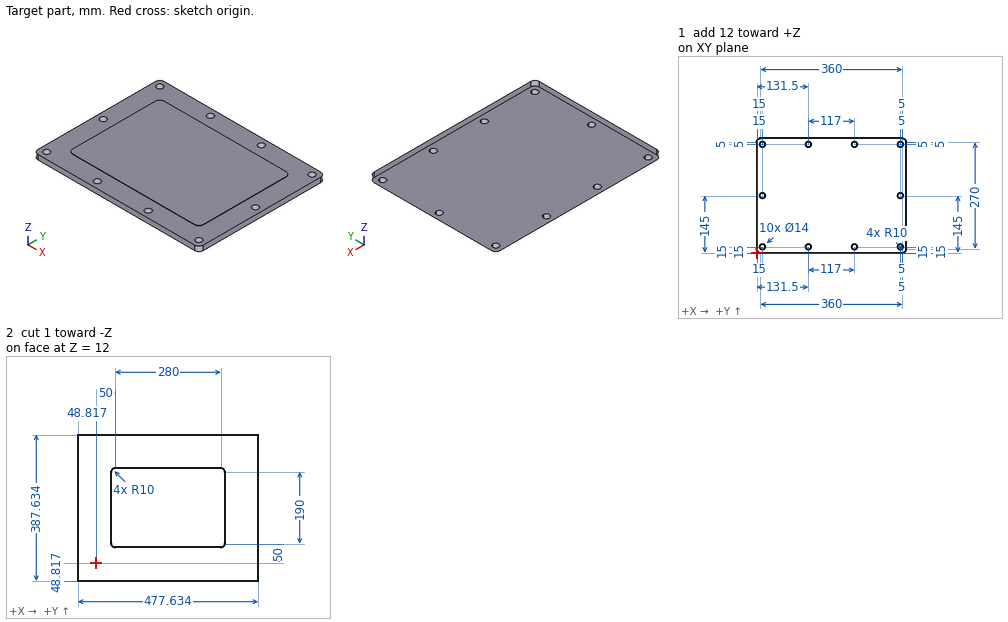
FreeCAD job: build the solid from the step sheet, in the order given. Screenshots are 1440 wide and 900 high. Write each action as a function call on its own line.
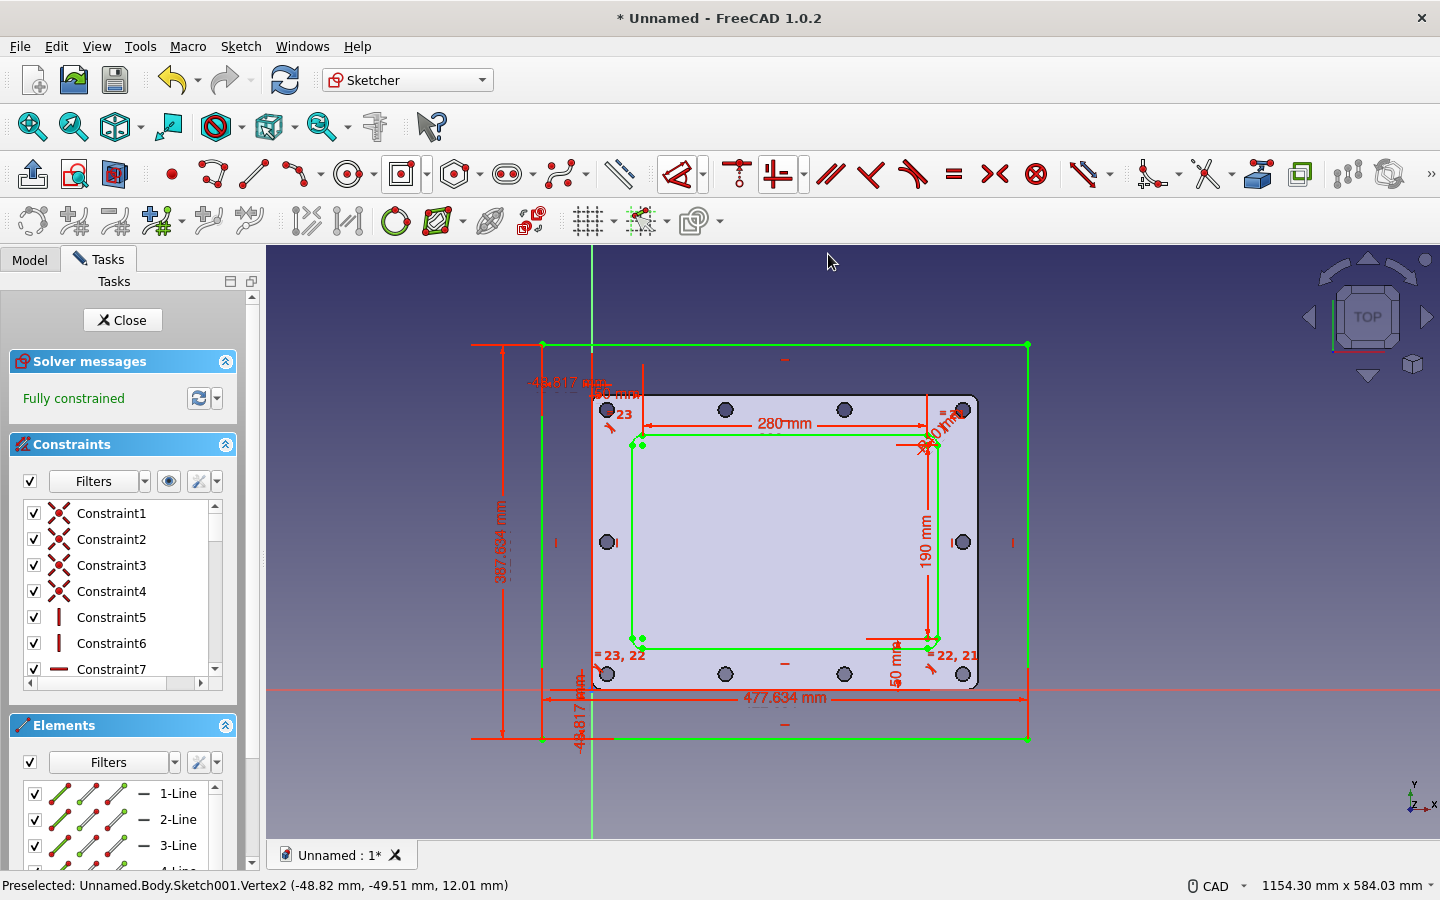
click(123, 320)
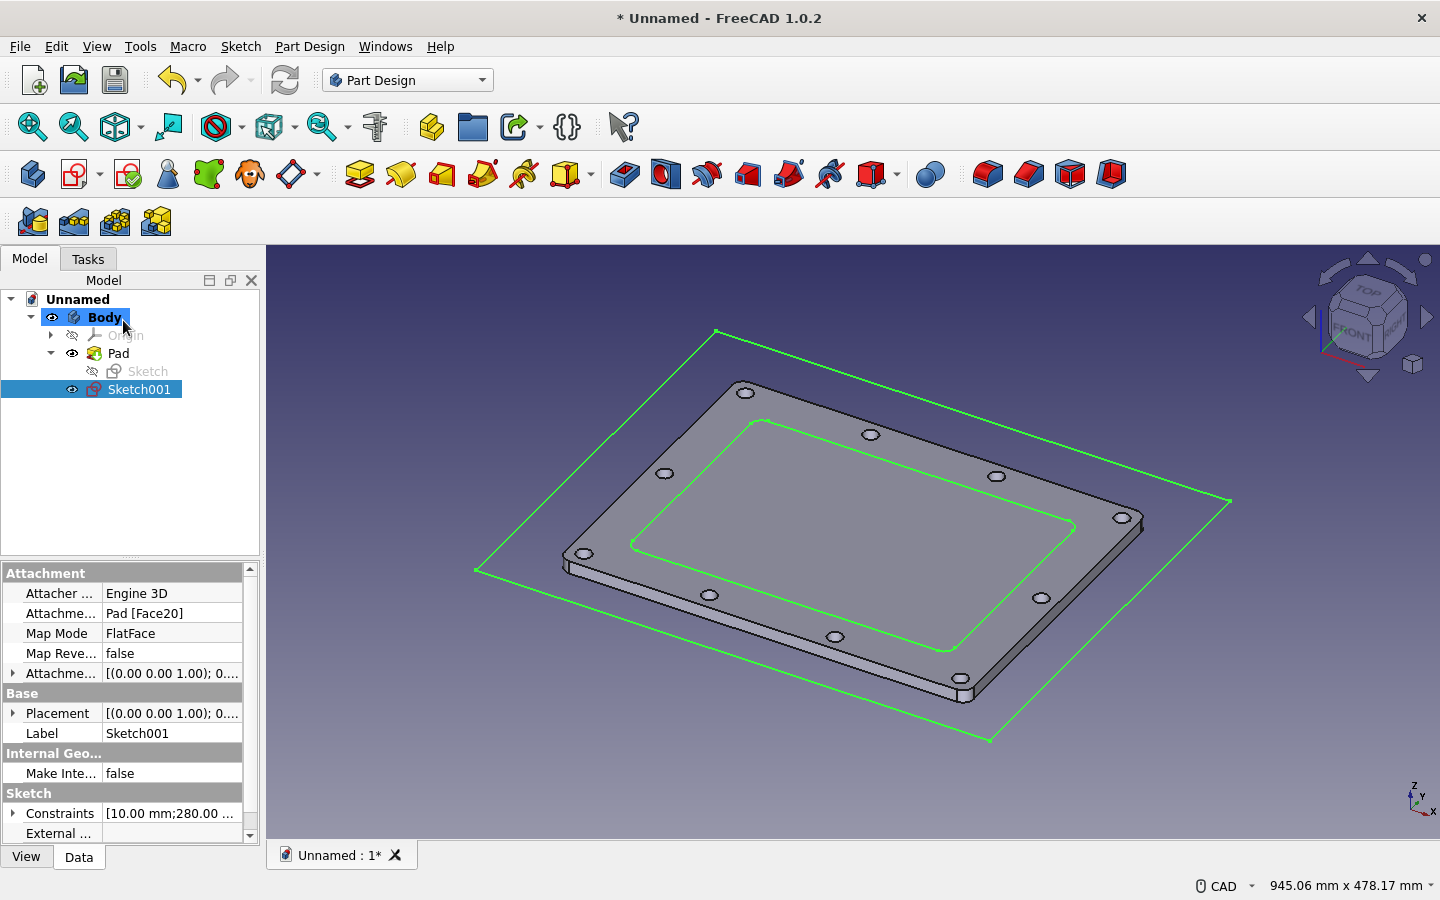
click(625, 174)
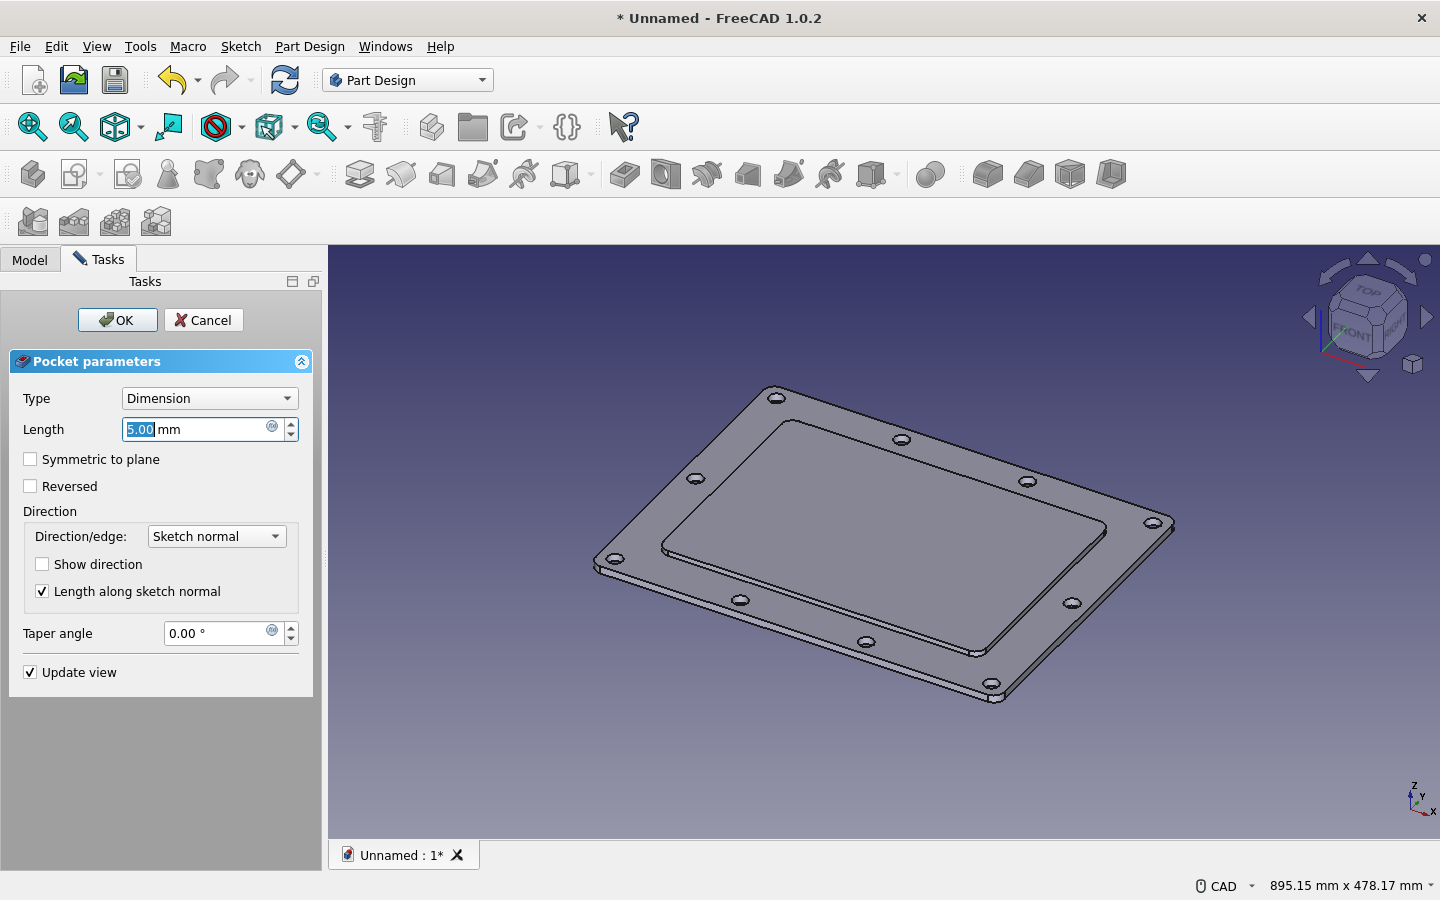
text(1)
key(Tab)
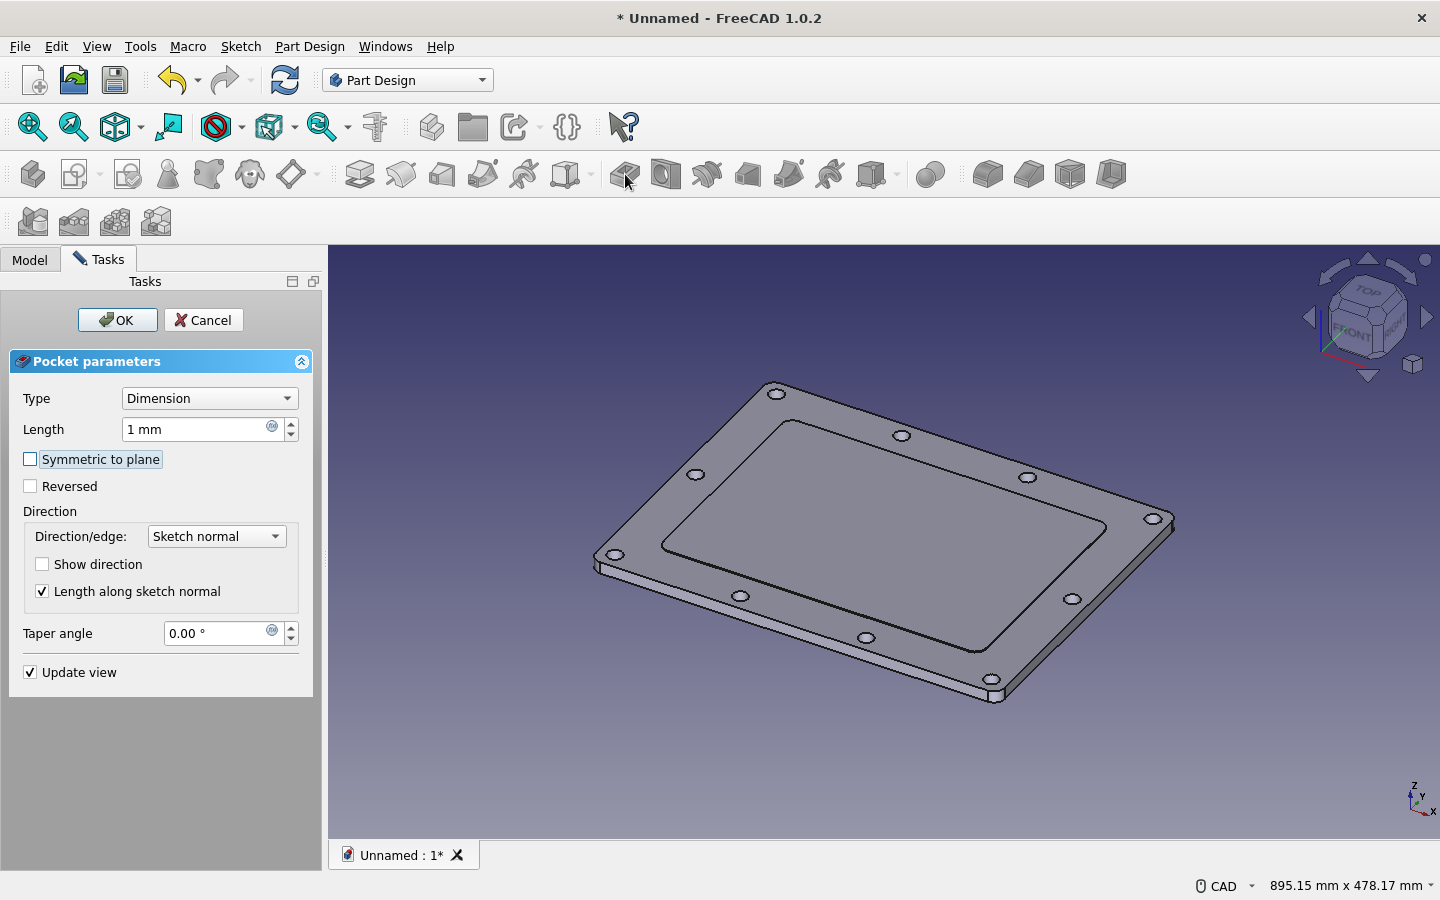
click(118, 320)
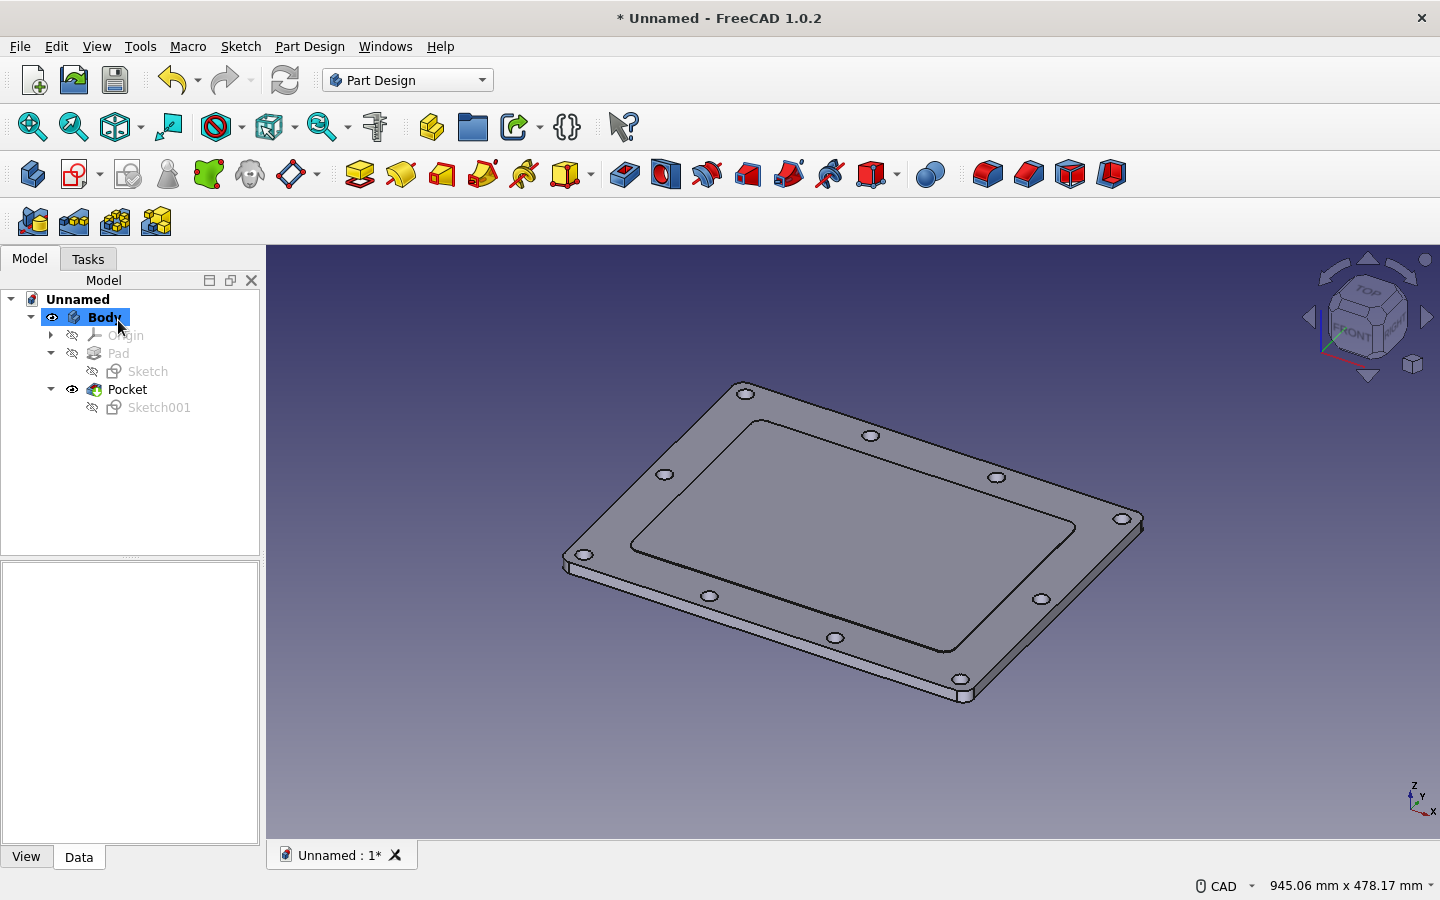
key(0)